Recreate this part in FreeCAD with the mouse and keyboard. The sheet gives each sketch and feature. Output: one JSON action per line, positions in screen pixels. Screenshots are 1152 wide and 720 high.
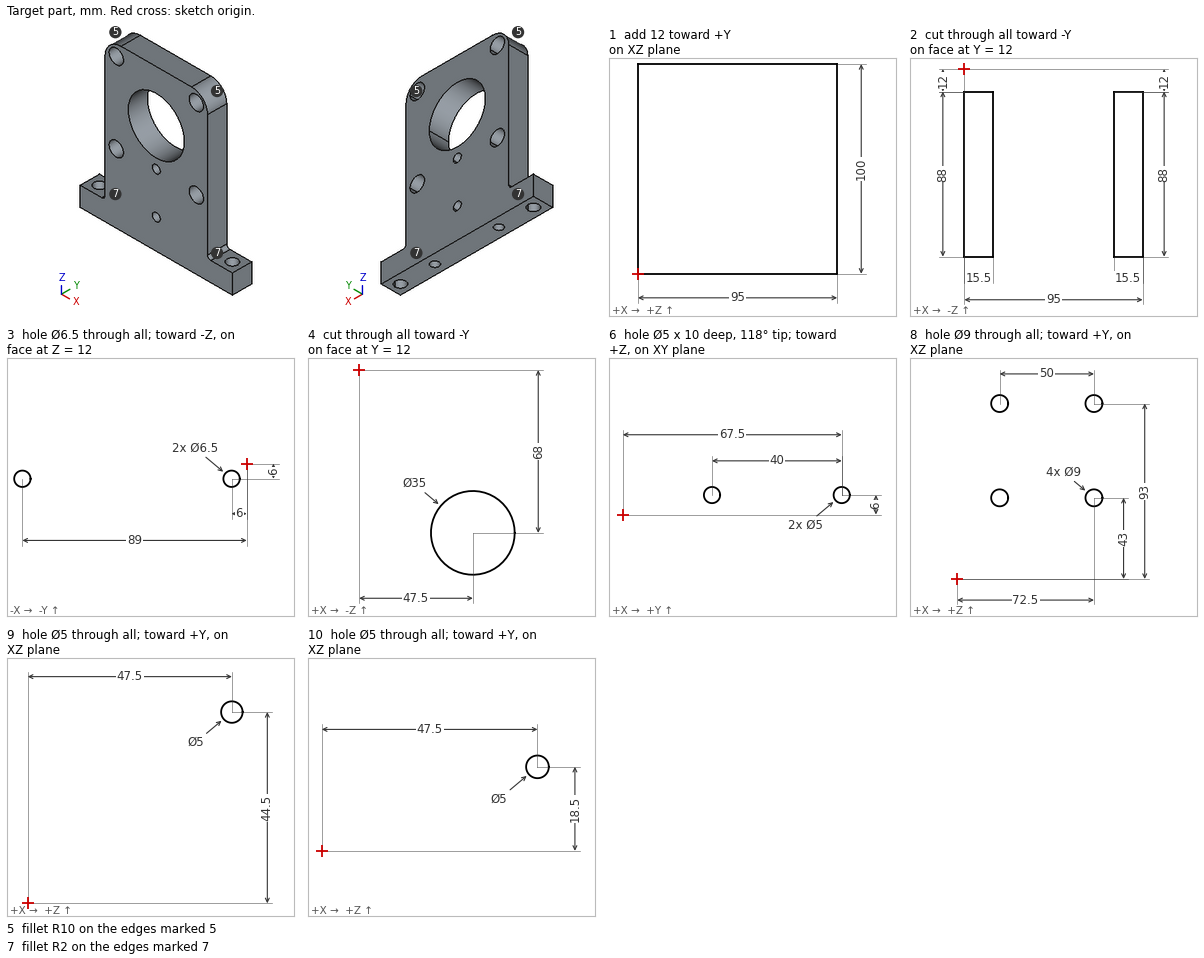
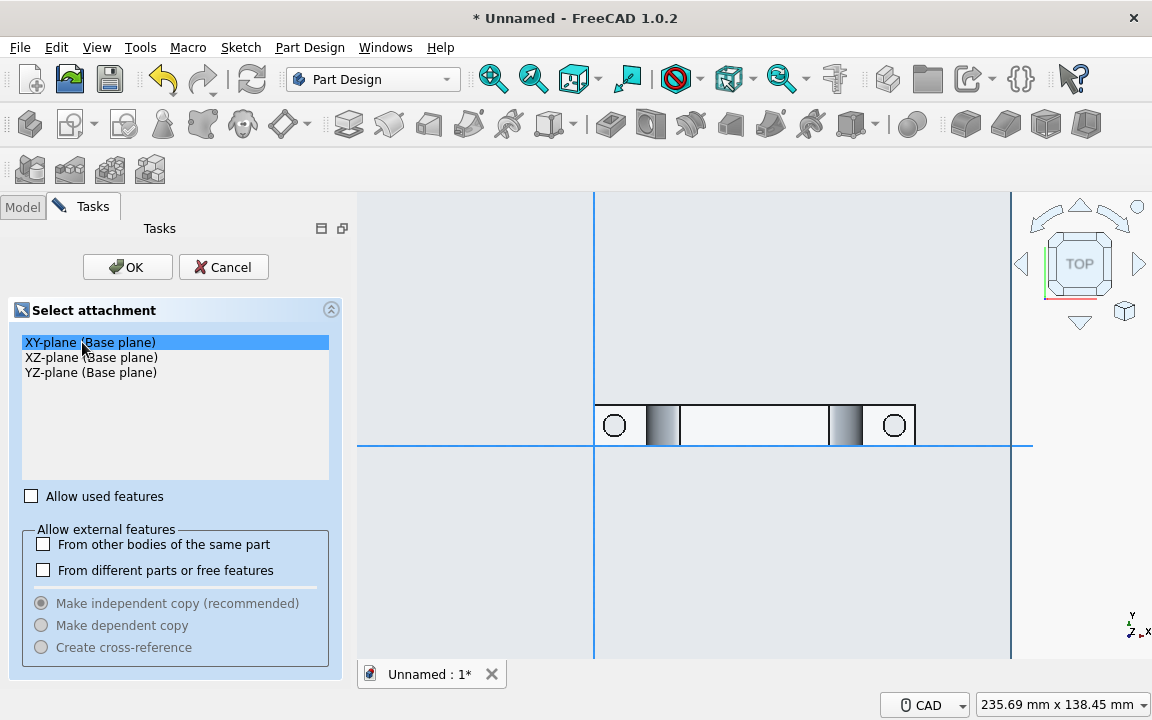
{"action": "left_click", "coordinate": [128, 267]}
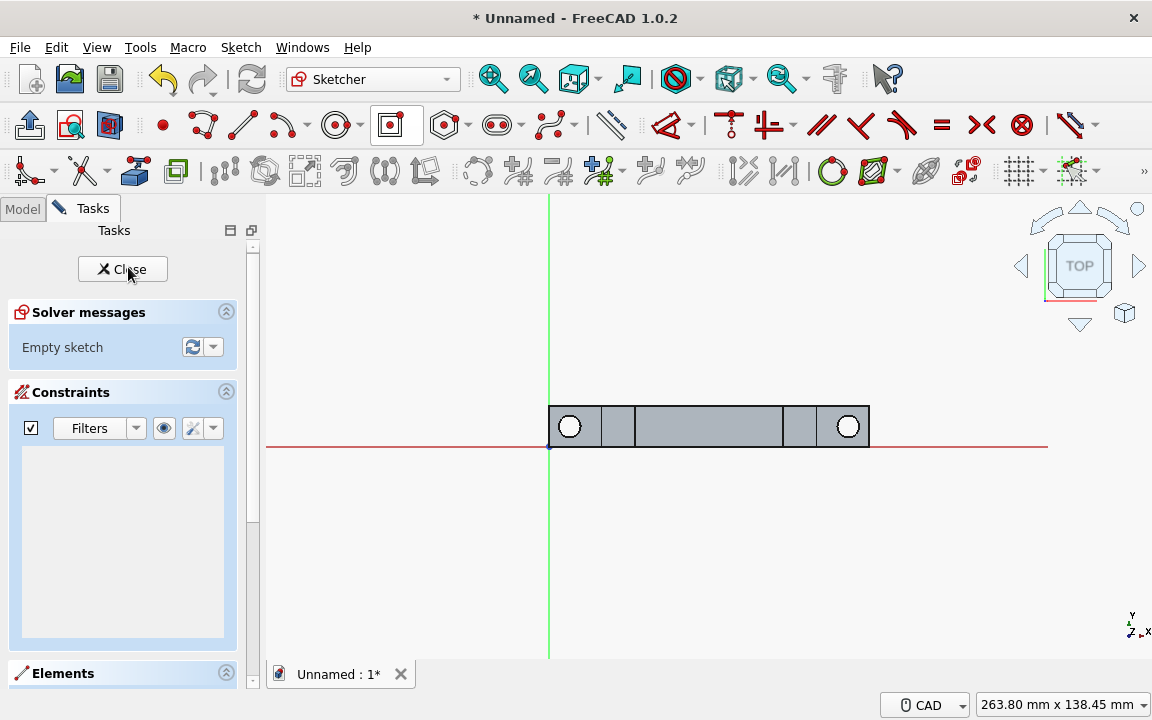
{"action": "left_click", "coordinate": [110, 126]}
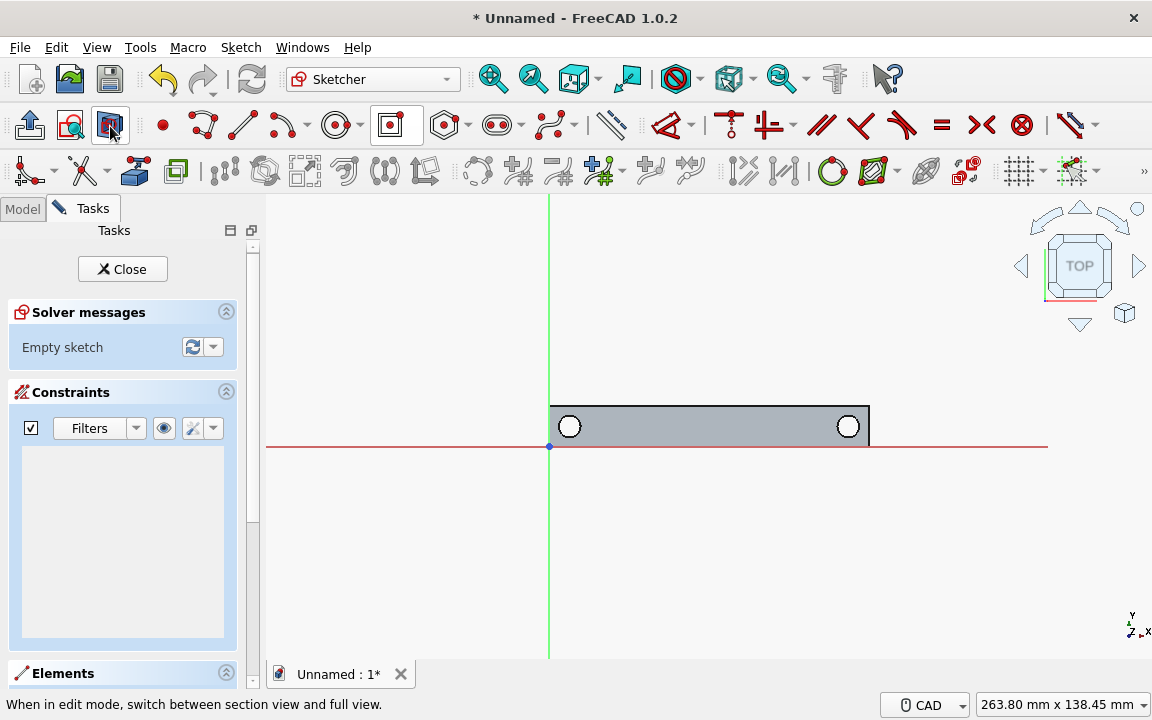
{"action": "scroll", "coordinate": [689, 437], "scroll_direction": "up", "scroll_amount": 4}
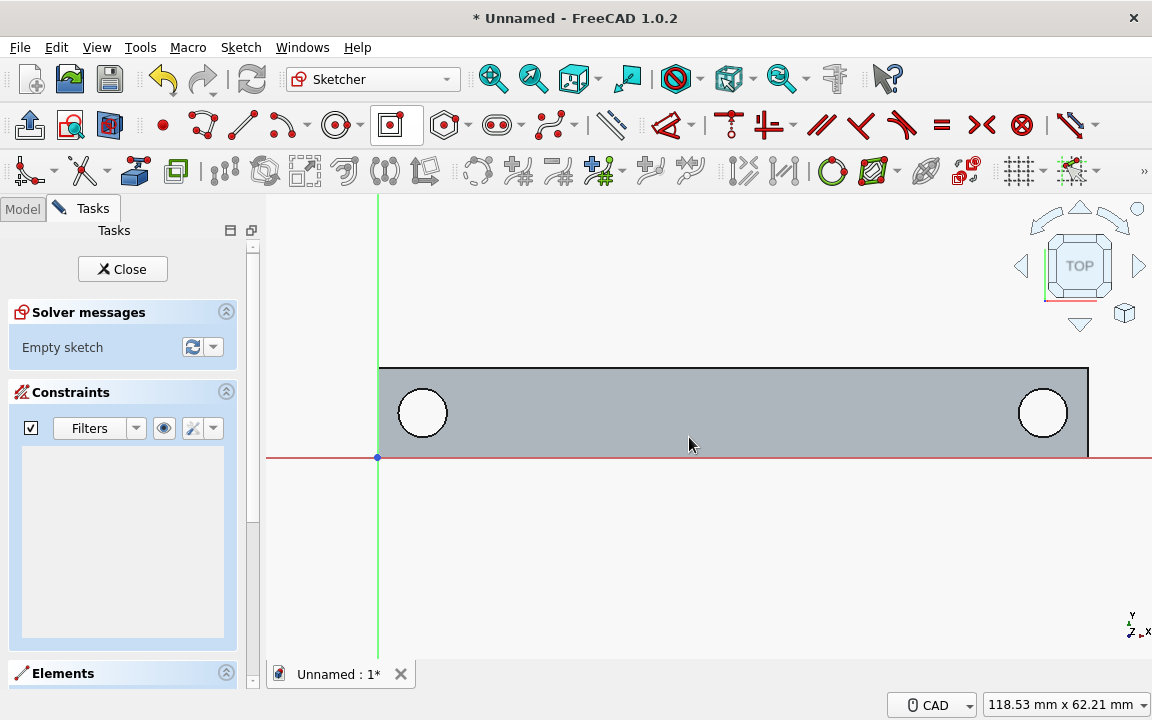
{"action": "left_click", "coordinate": [336, 126]}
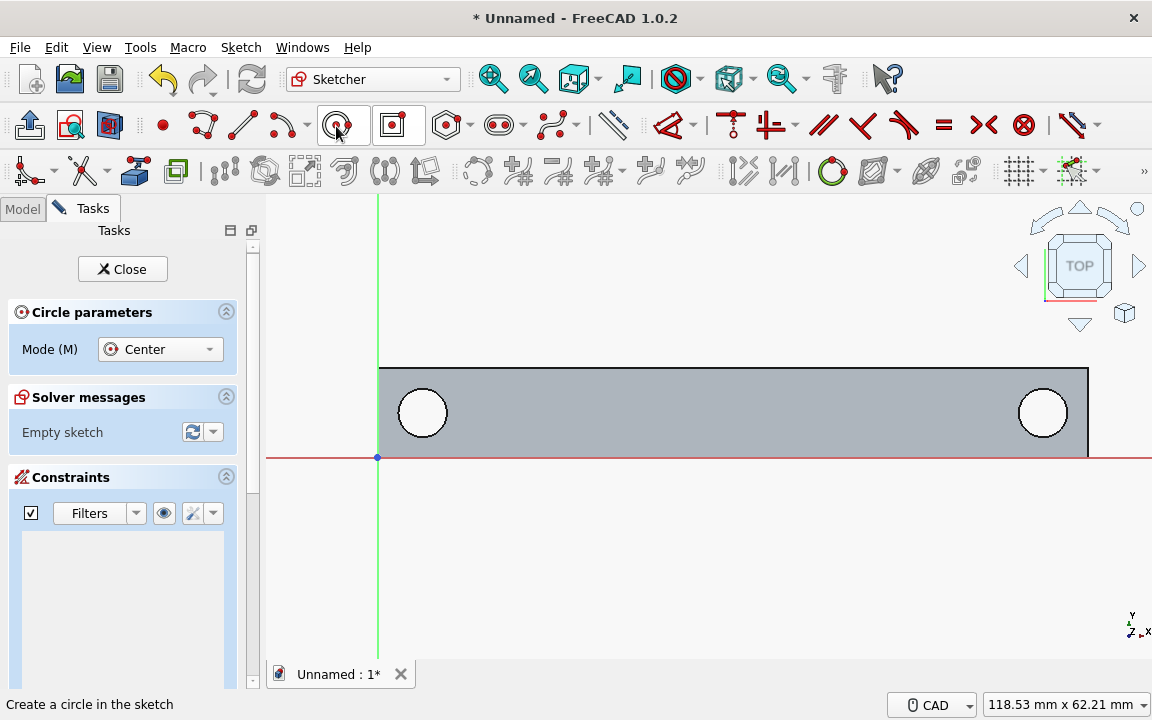
{"action": "left_click", "coordinate": [882, 413]}
{"action": "left_click", "coordinate": [896, 400]}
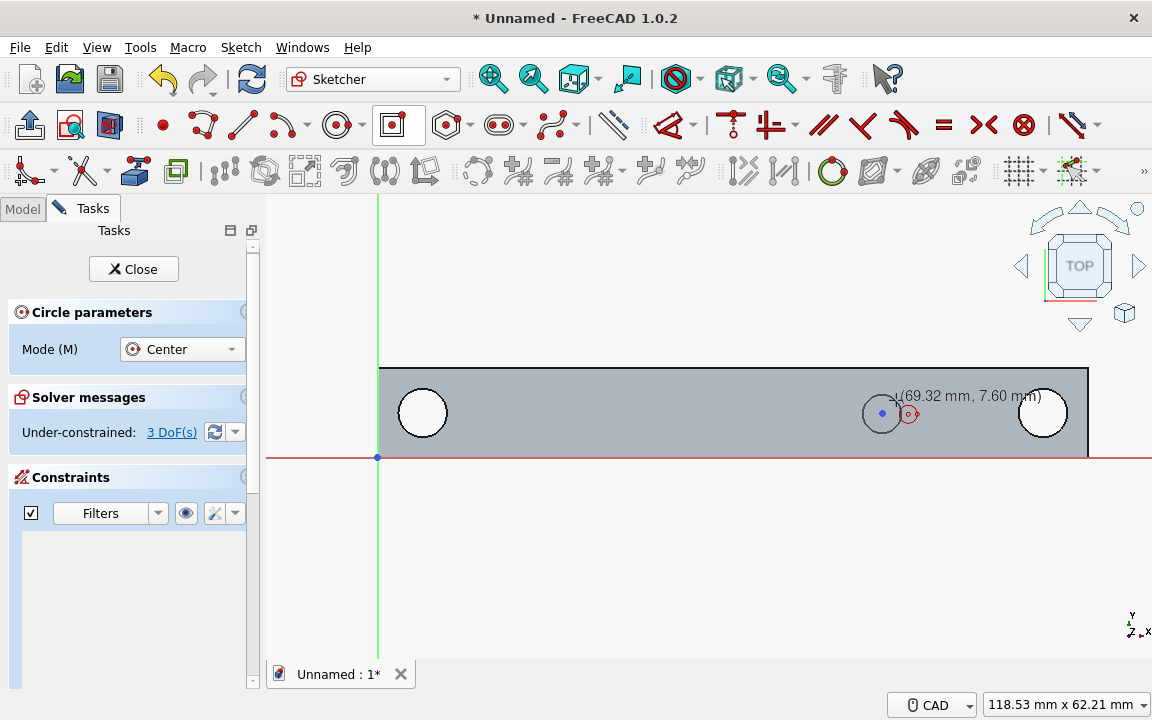
{"action": "left_click", "coordinate": [583, 413]}
{"action": "left_click", "coordinate": [597, 400]}
{"action": "key", "text": "Escape"}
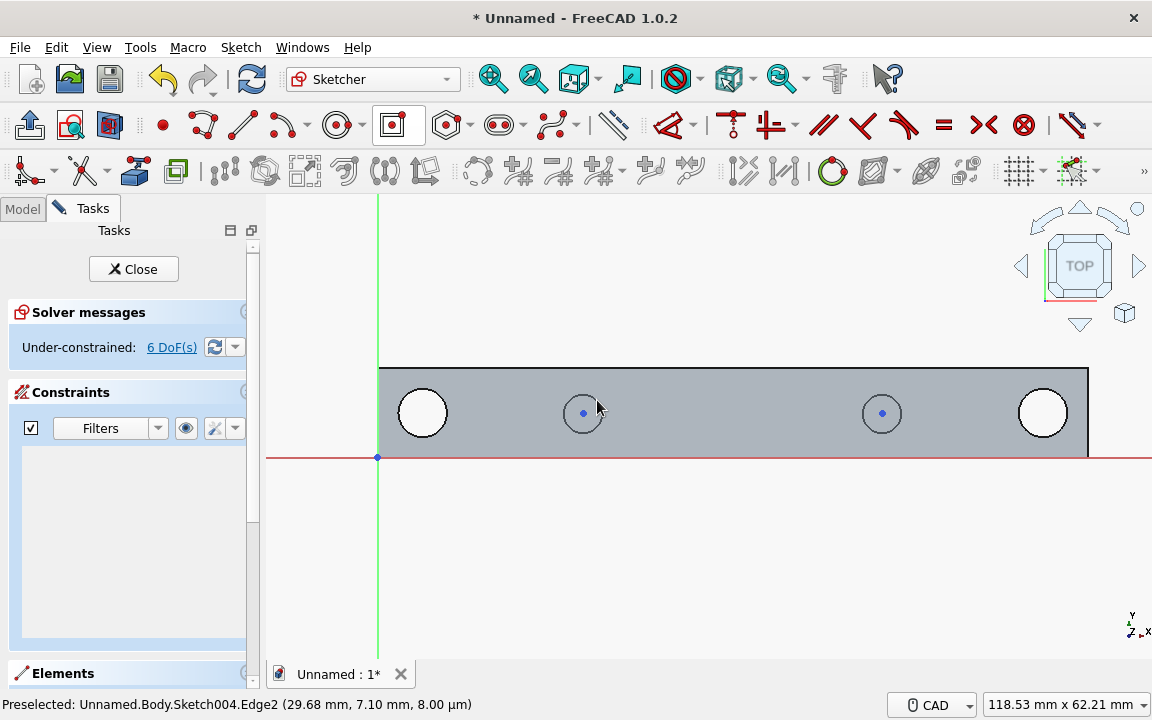
{"action": "left_click", "coordinate": [895, 400]}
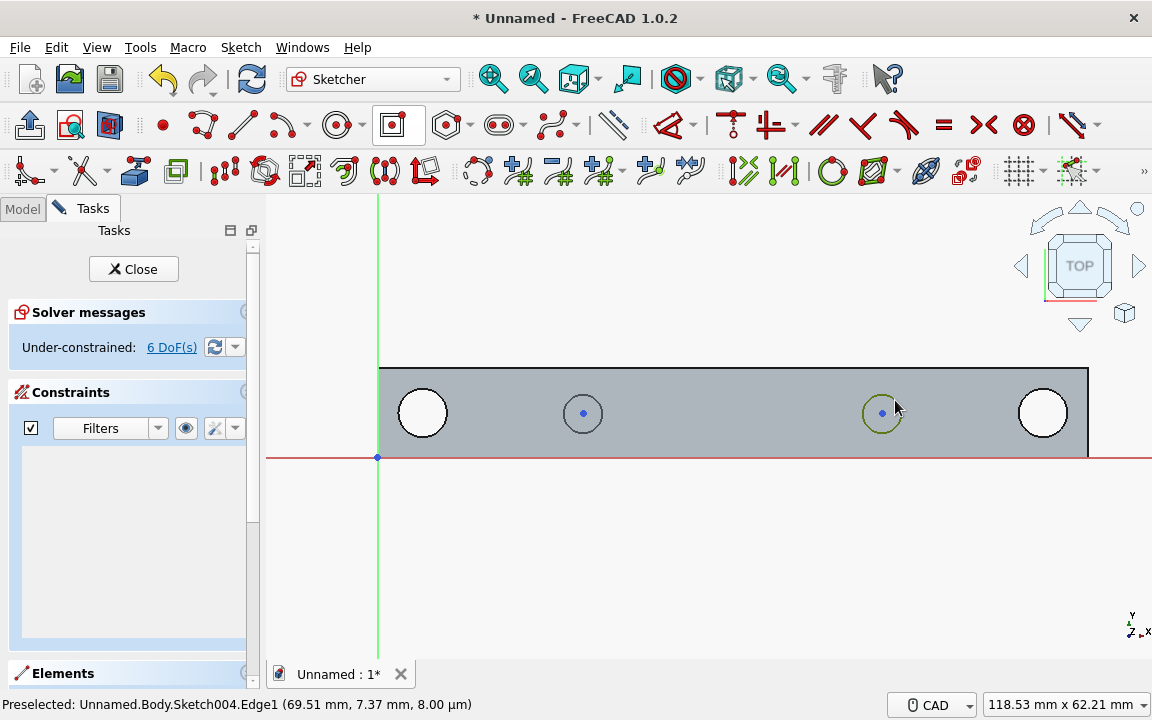
{"action": "left_click", "coordinate": [596, 400]}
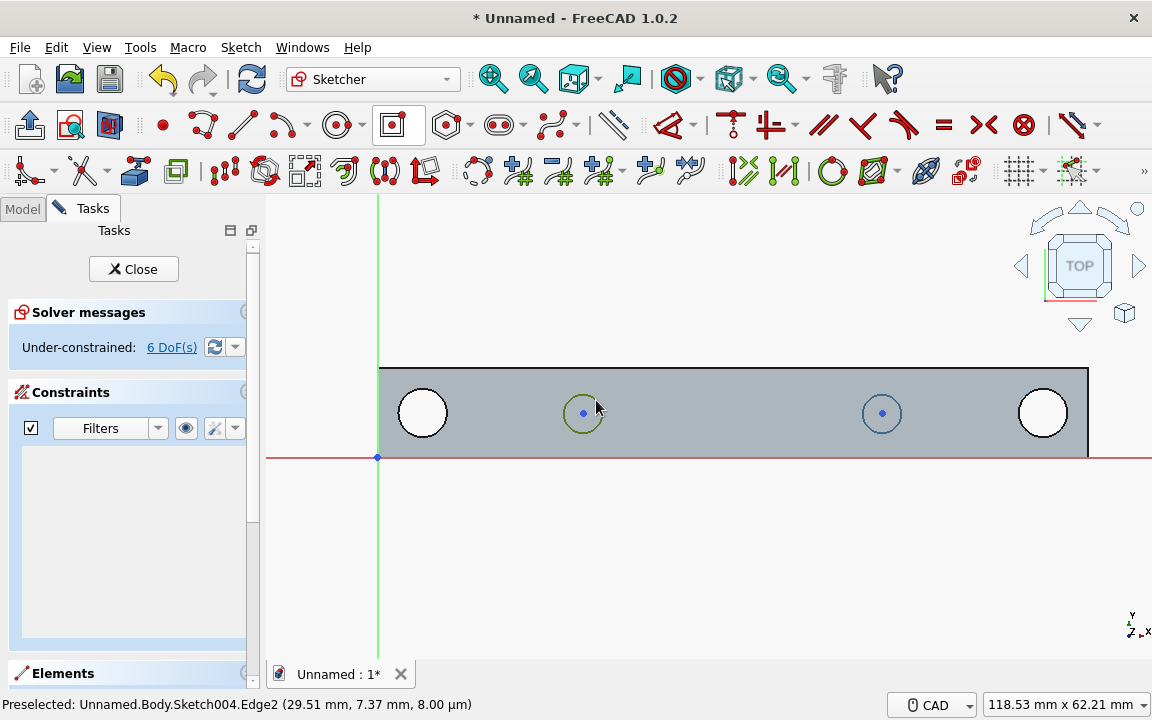
{"action": "left_click", "coordinate": [944, 126]}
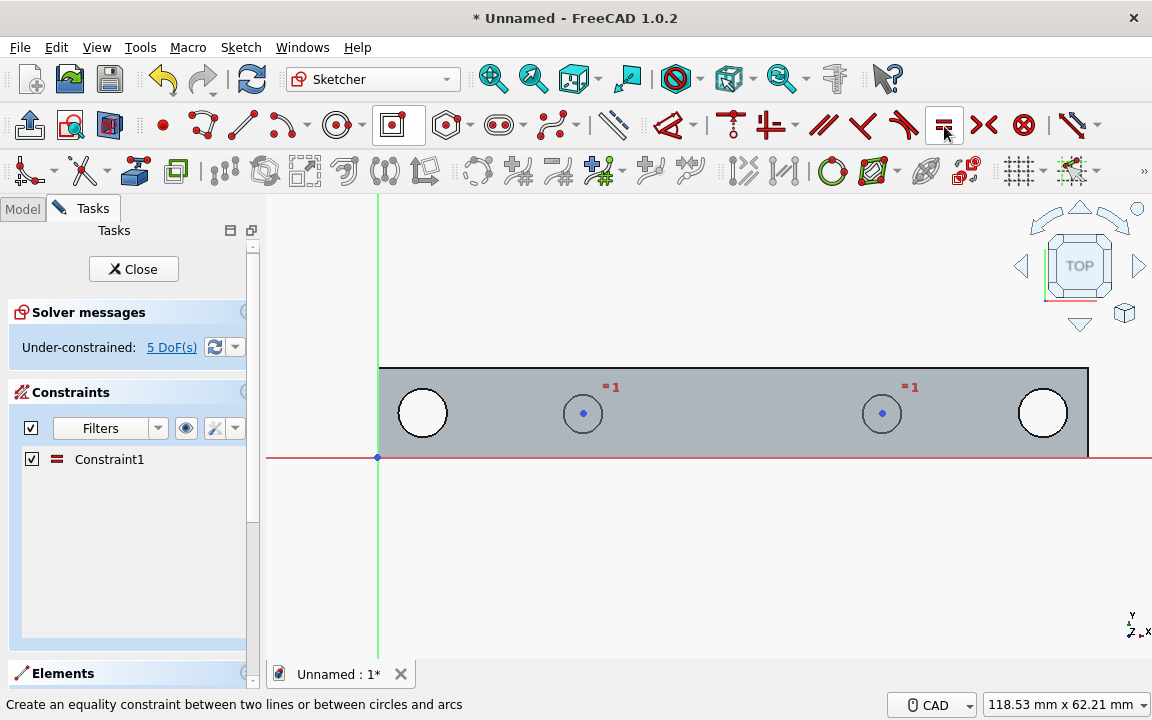
{"action": "left_click", "coordinate": [882, 414]}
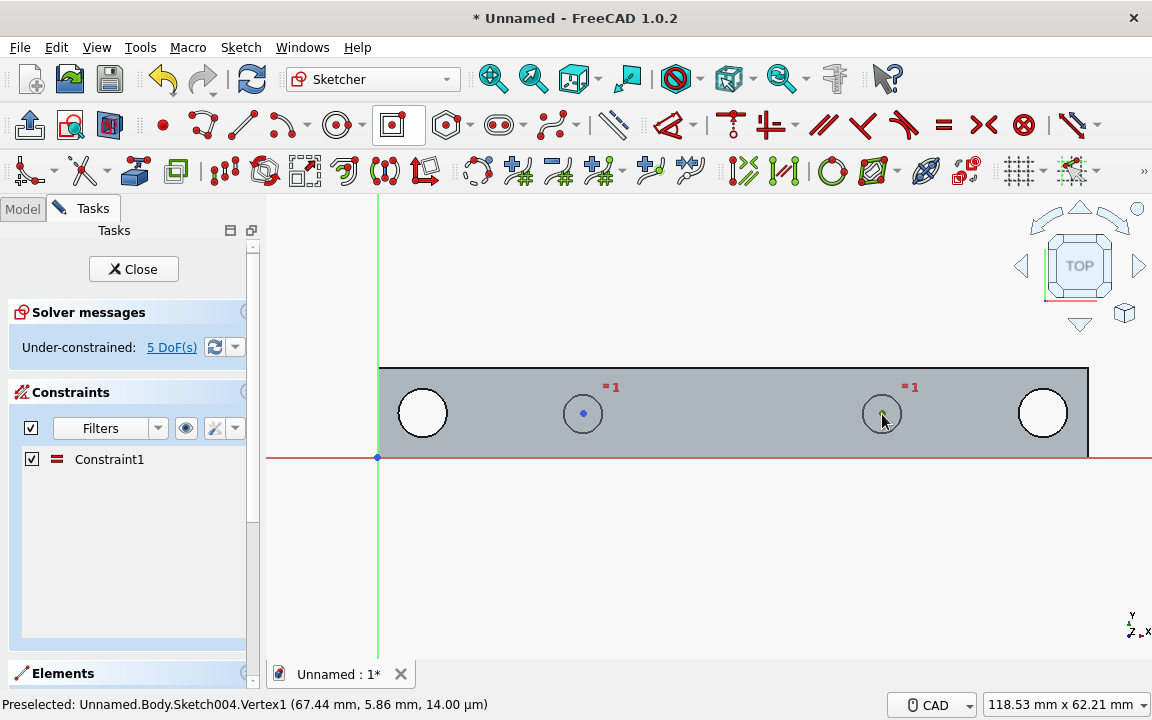
{"action": "left_click", "coordinate": [583, 414]}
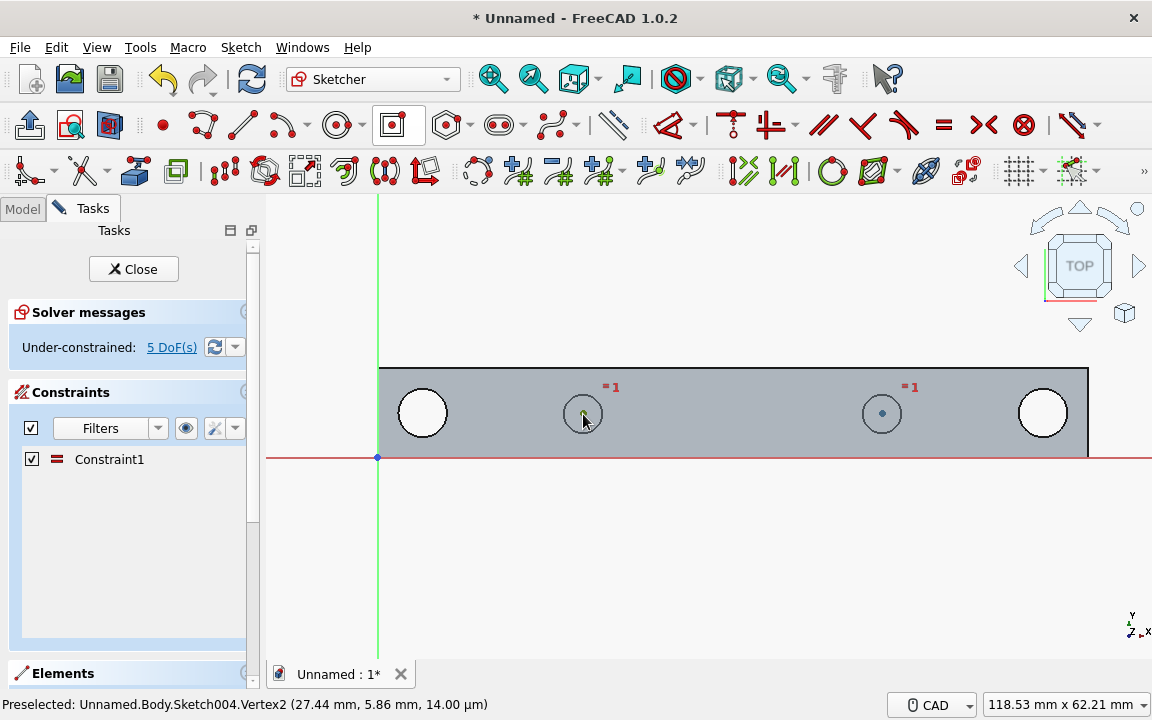
{"action": "key", "text": "h"}